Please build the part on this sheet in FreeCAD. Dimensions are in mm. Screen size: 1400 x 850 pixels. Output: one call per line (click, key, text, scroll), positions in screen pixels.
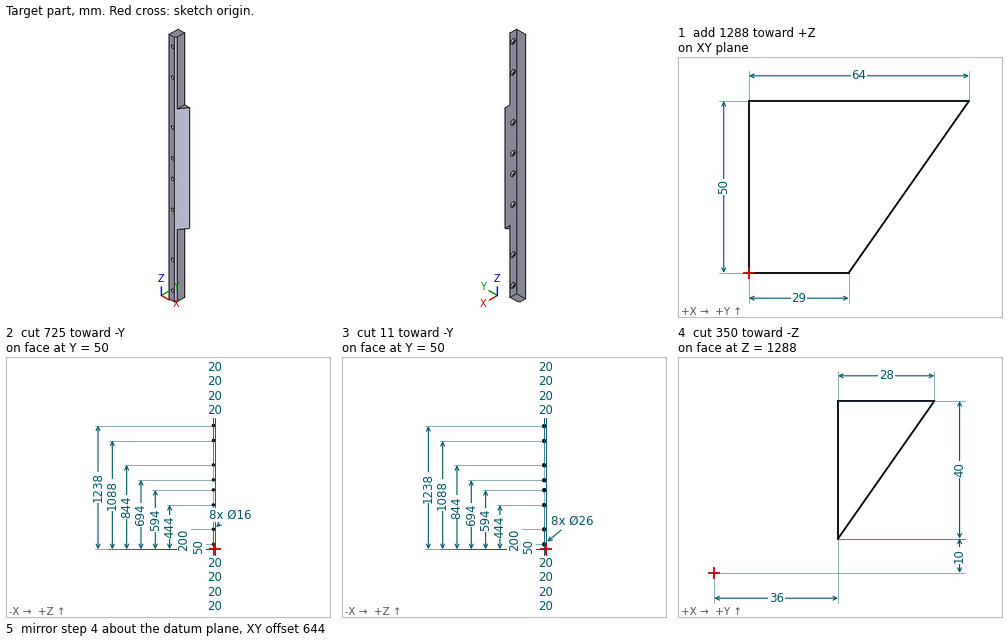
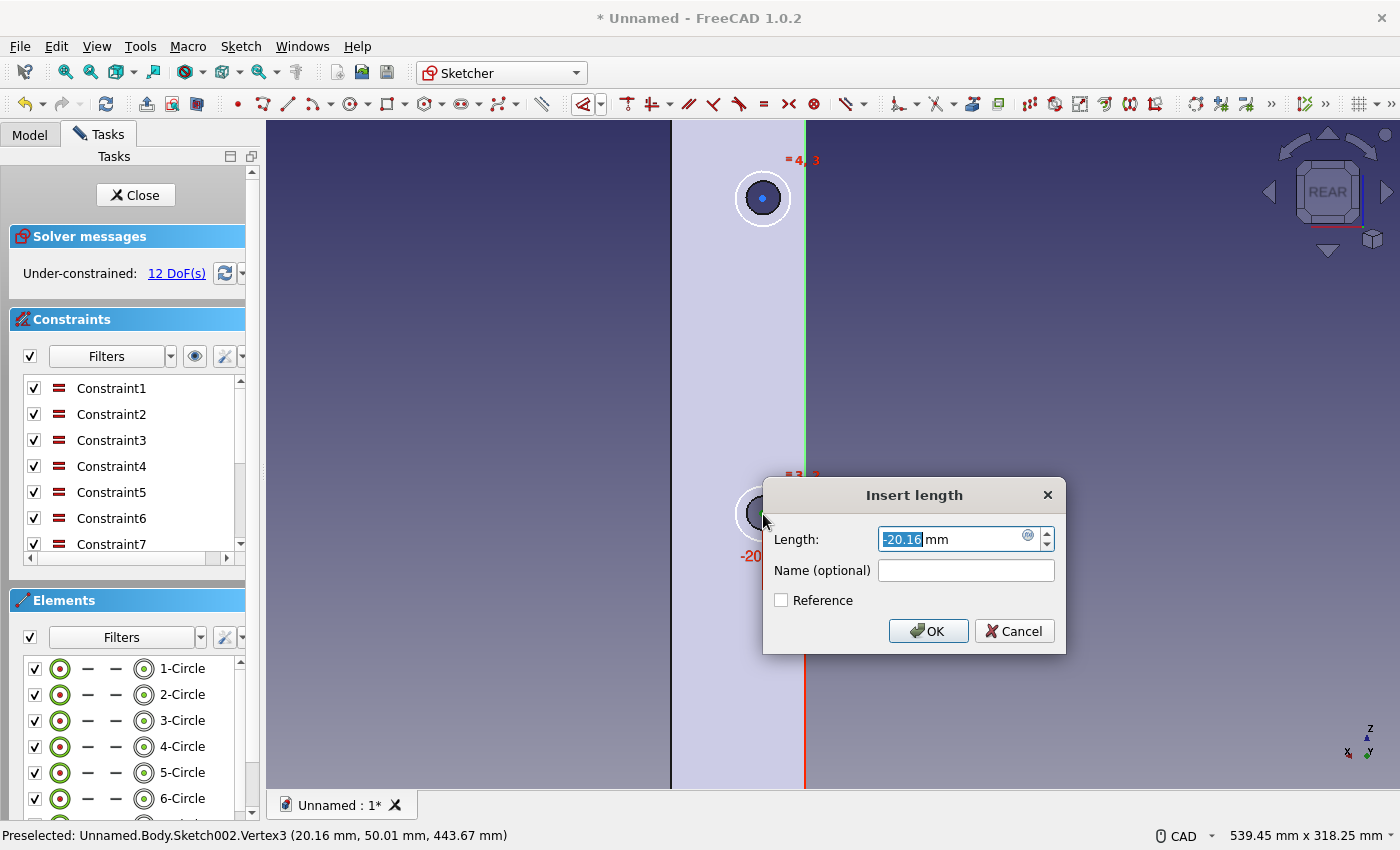
text(-20)
key(Return)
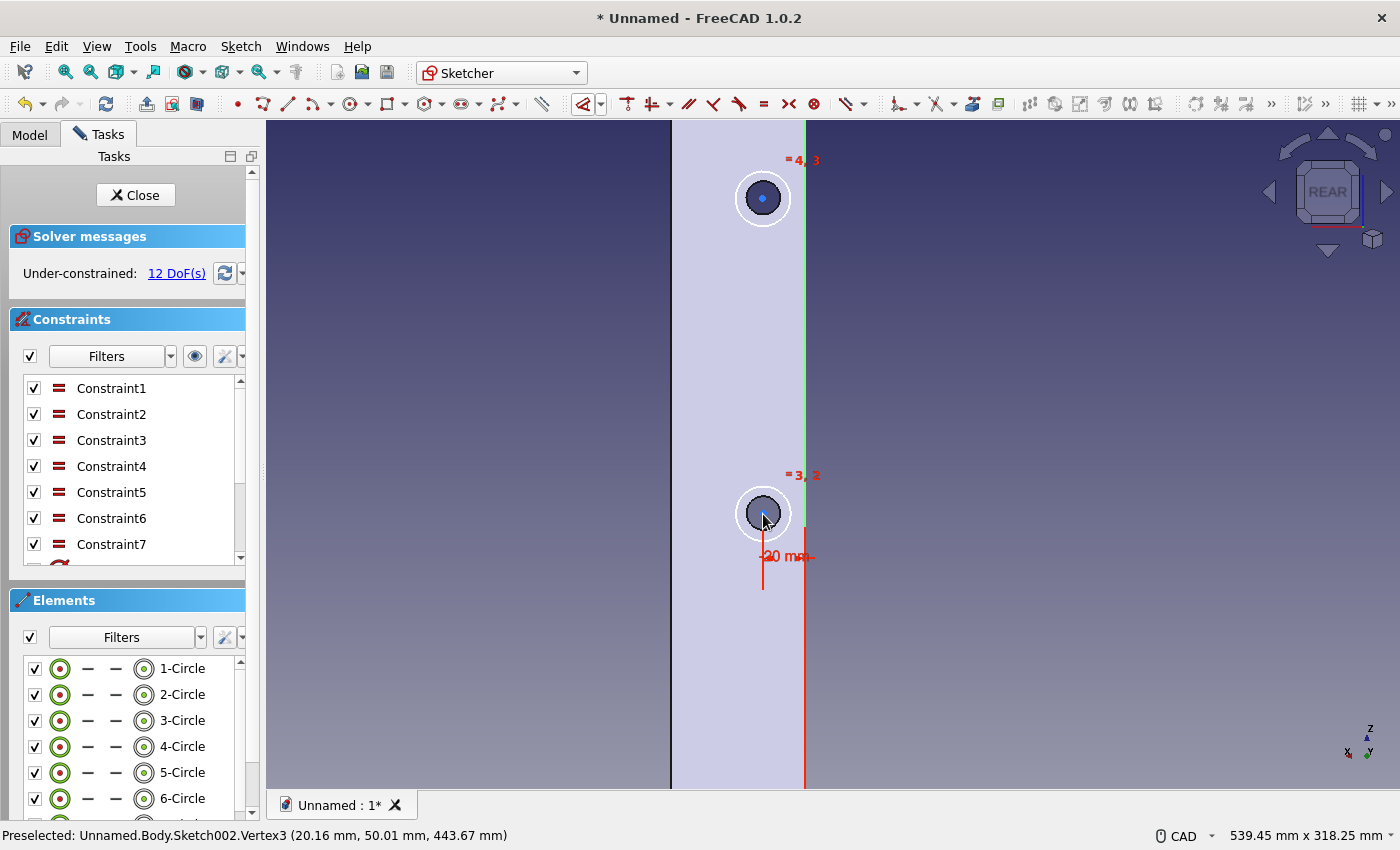
click(763, 199)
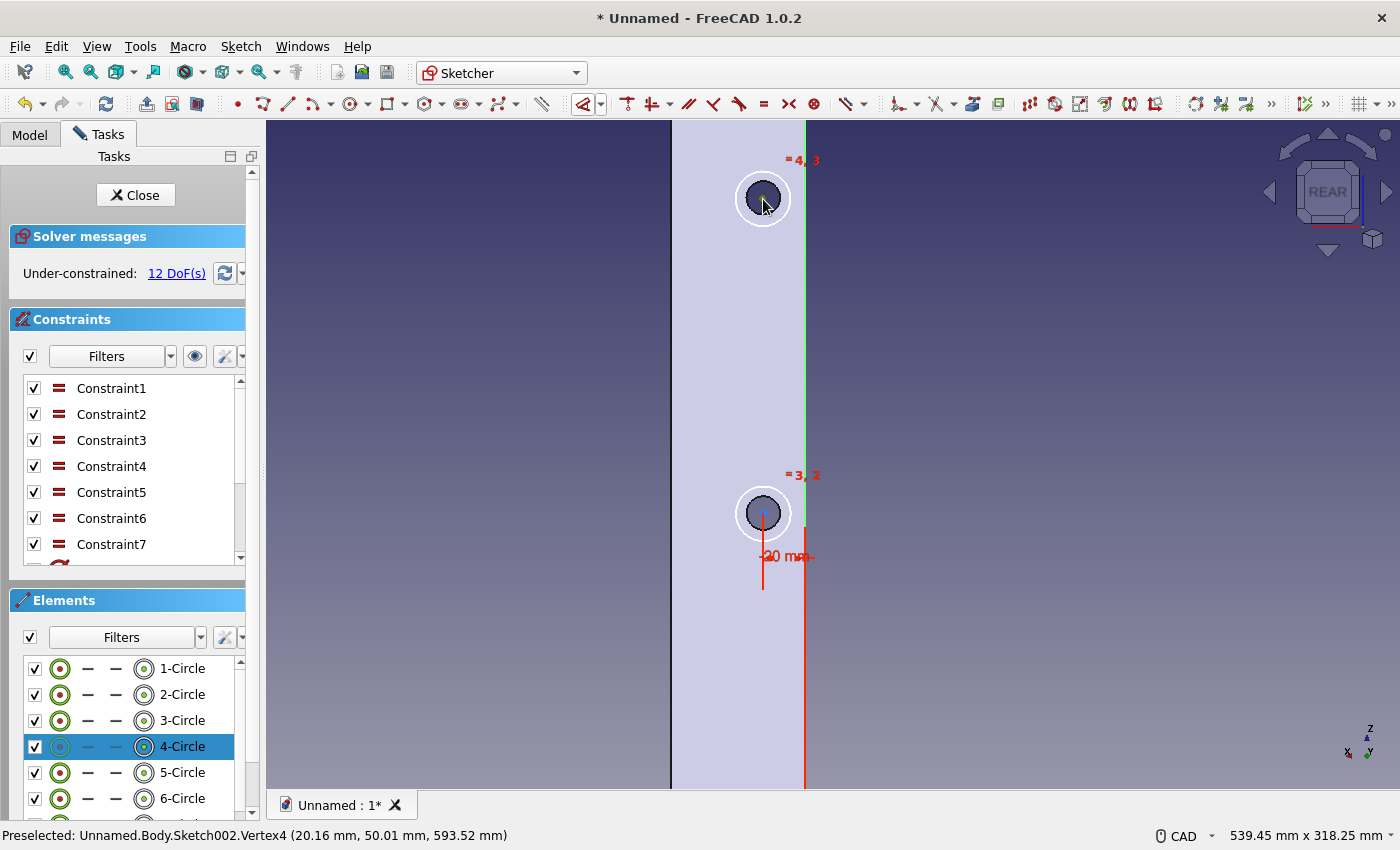
key(l)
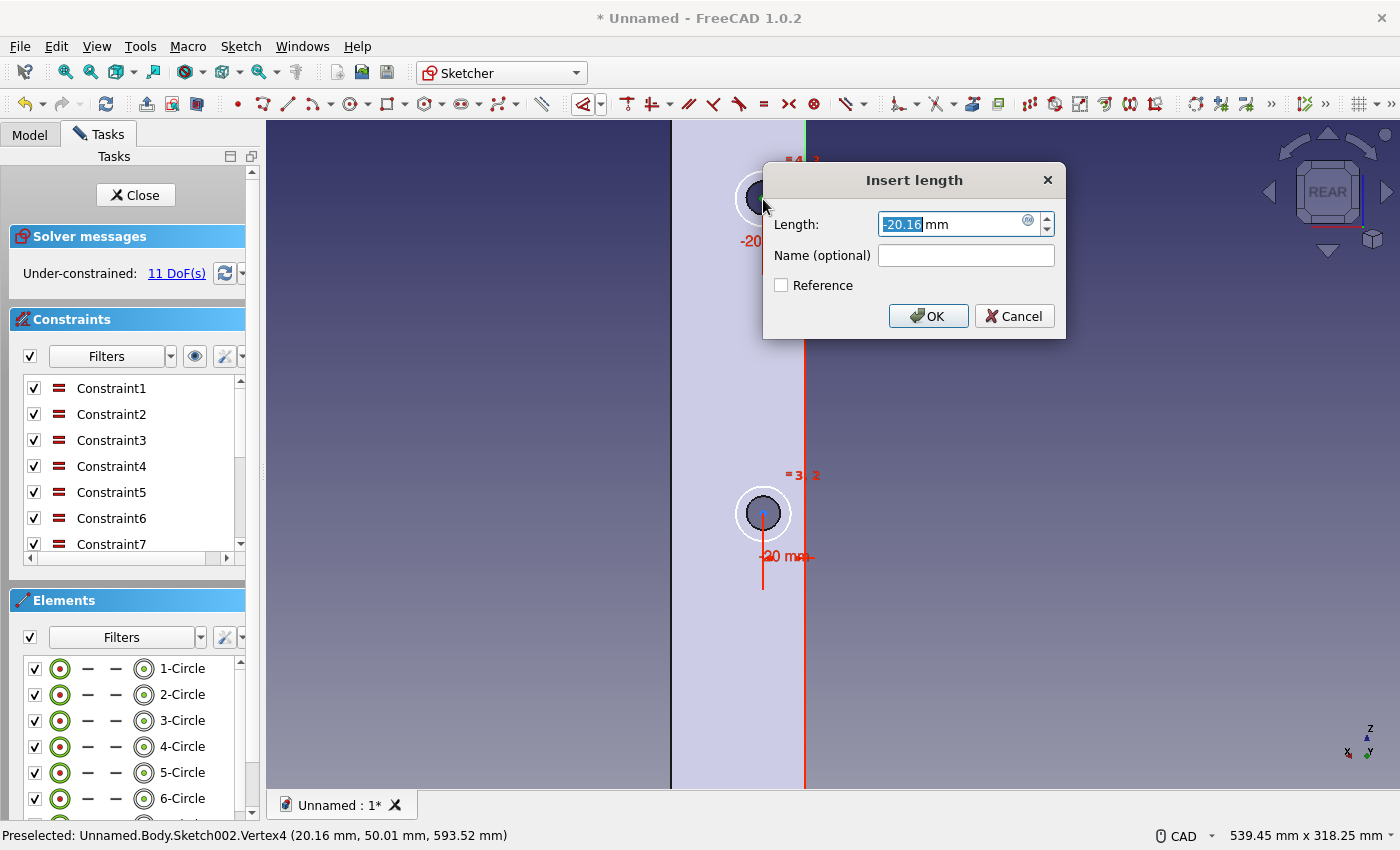
text(-20)
key(Return)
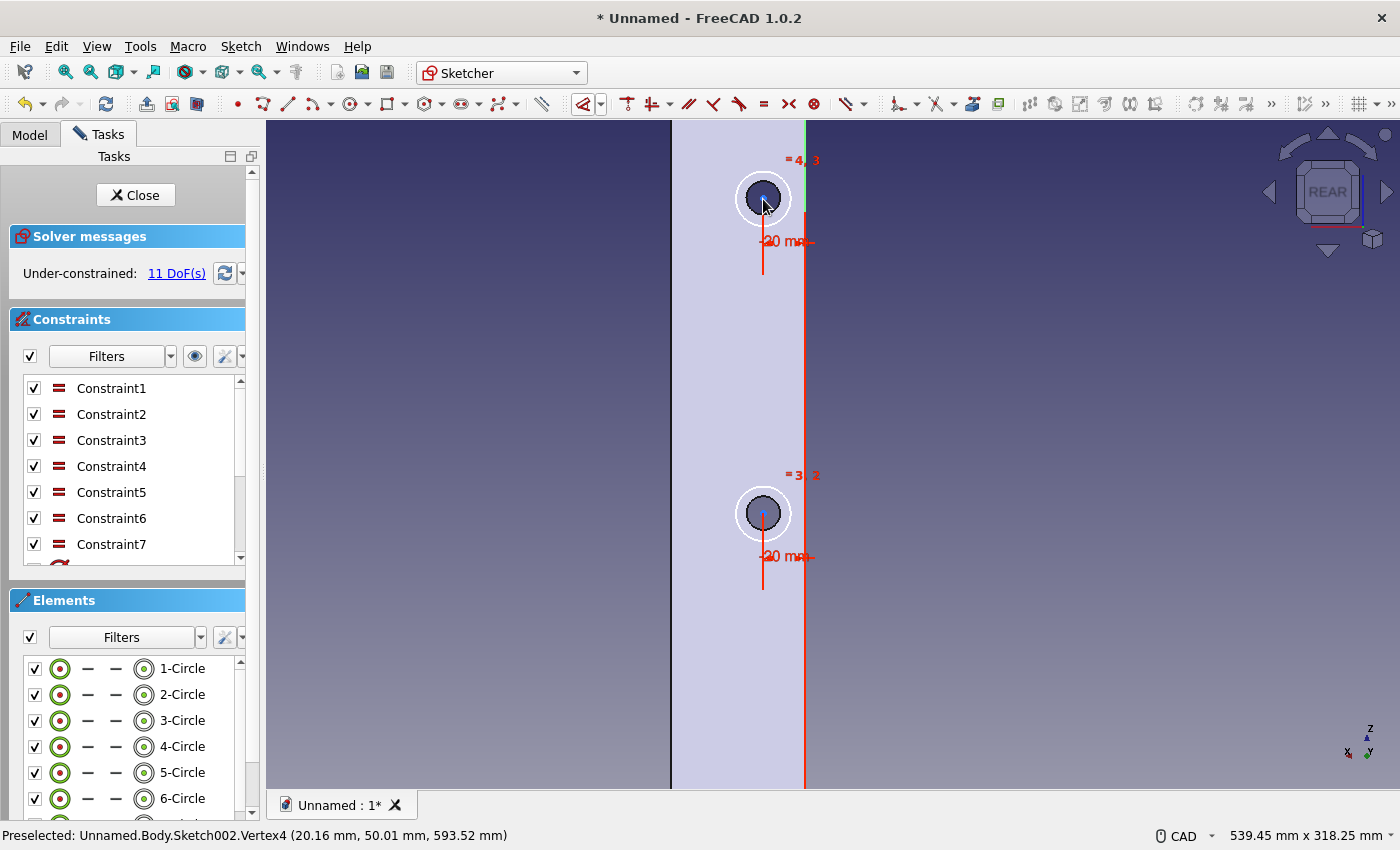
scroll(763, 518, down, 9)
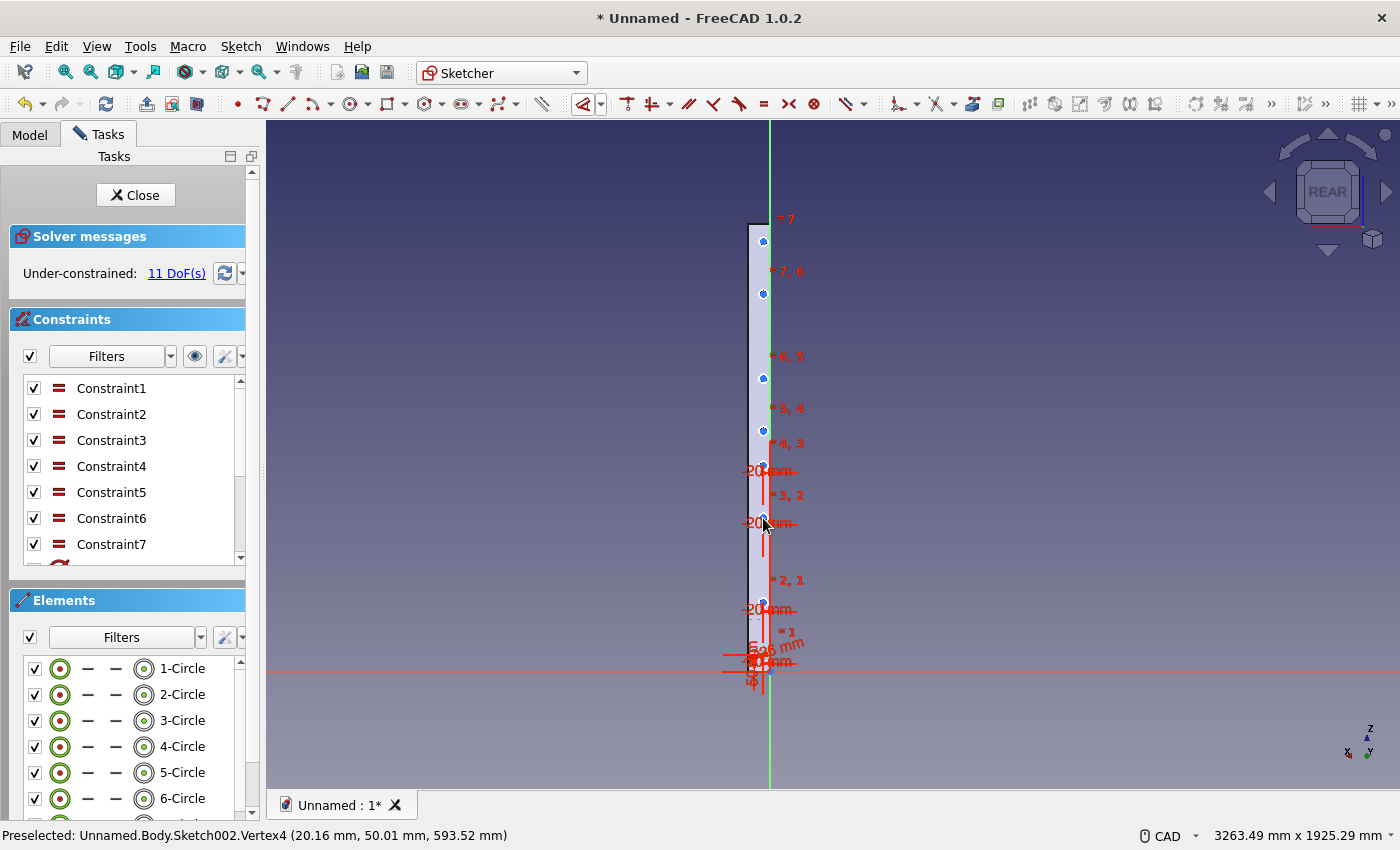
scroll(763, 431, up, 9)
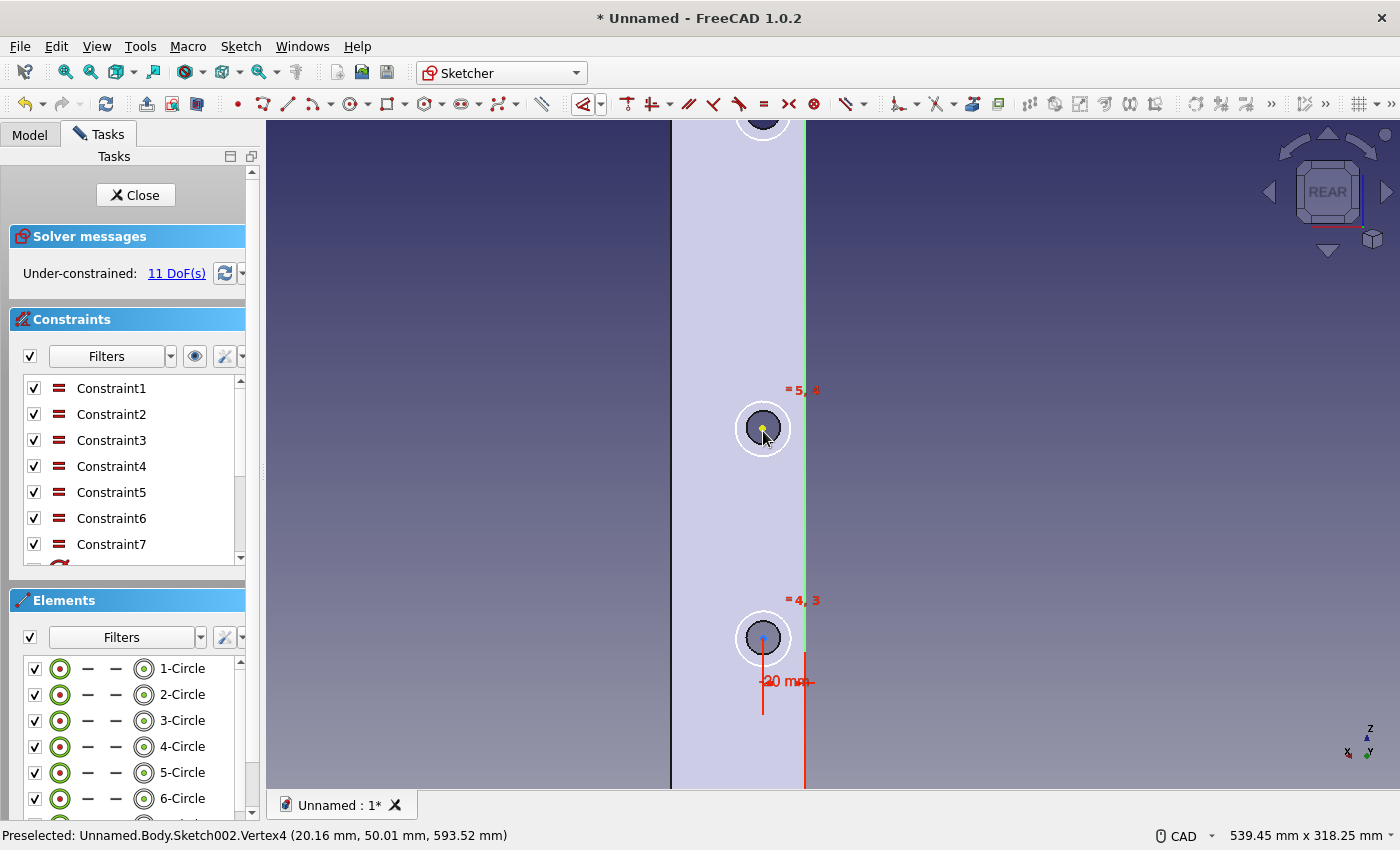
click(763, 429)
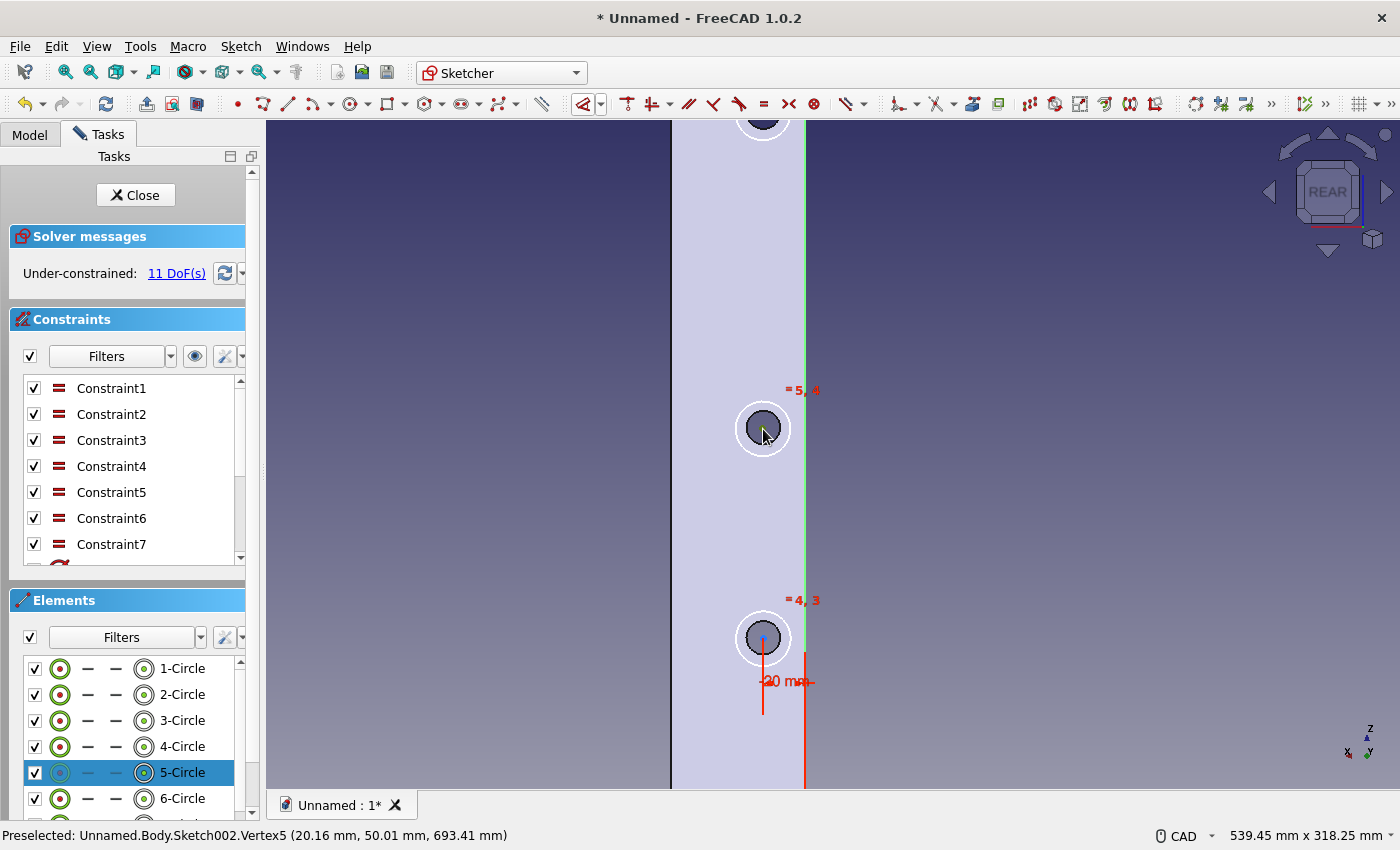
key(l)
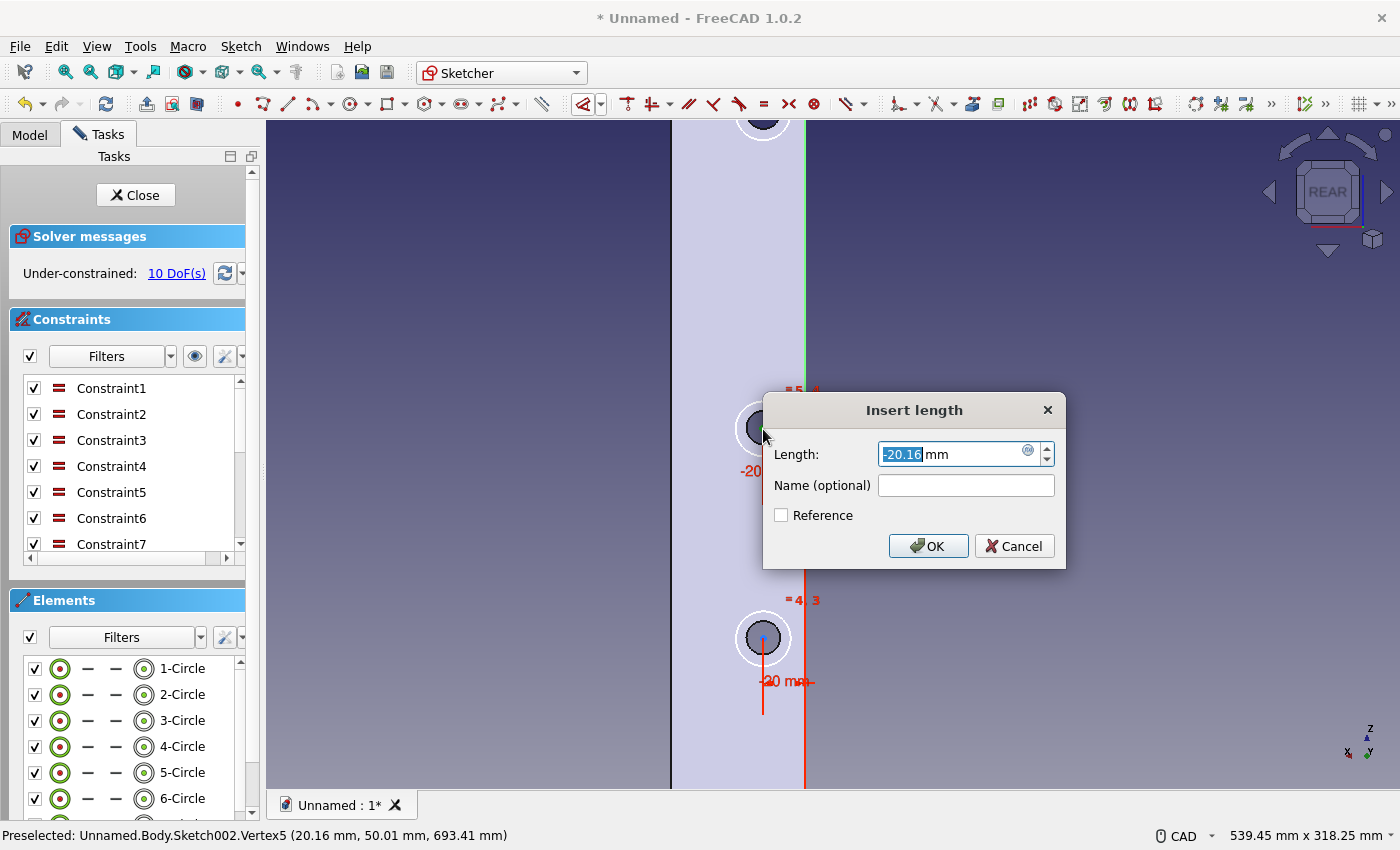
text(-20)
key(Return)